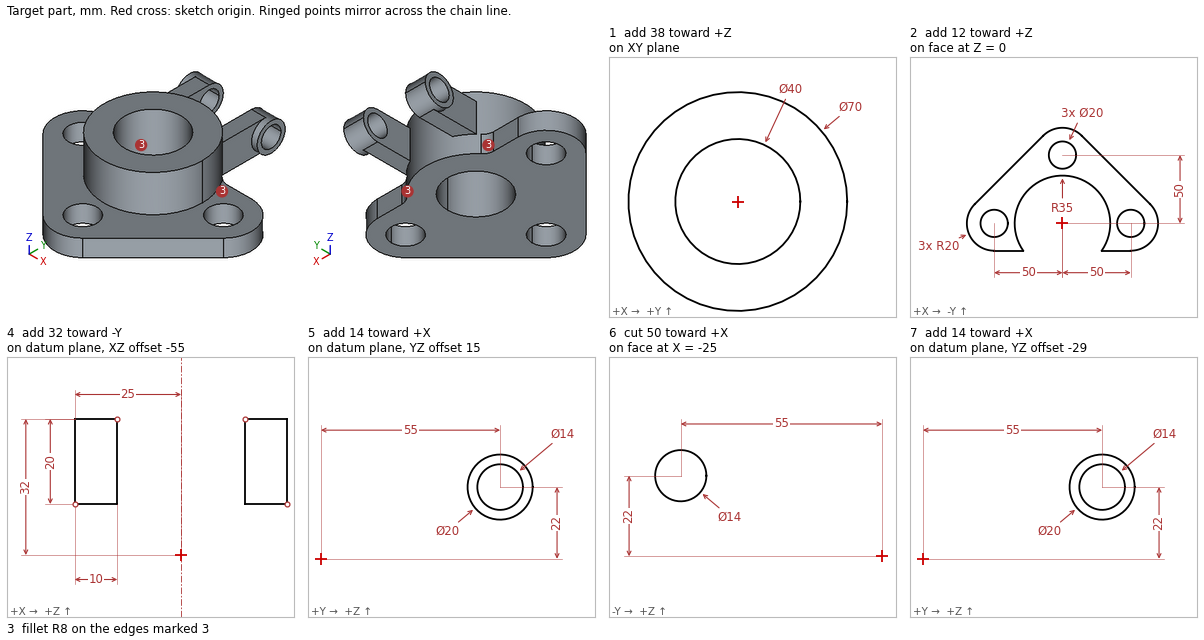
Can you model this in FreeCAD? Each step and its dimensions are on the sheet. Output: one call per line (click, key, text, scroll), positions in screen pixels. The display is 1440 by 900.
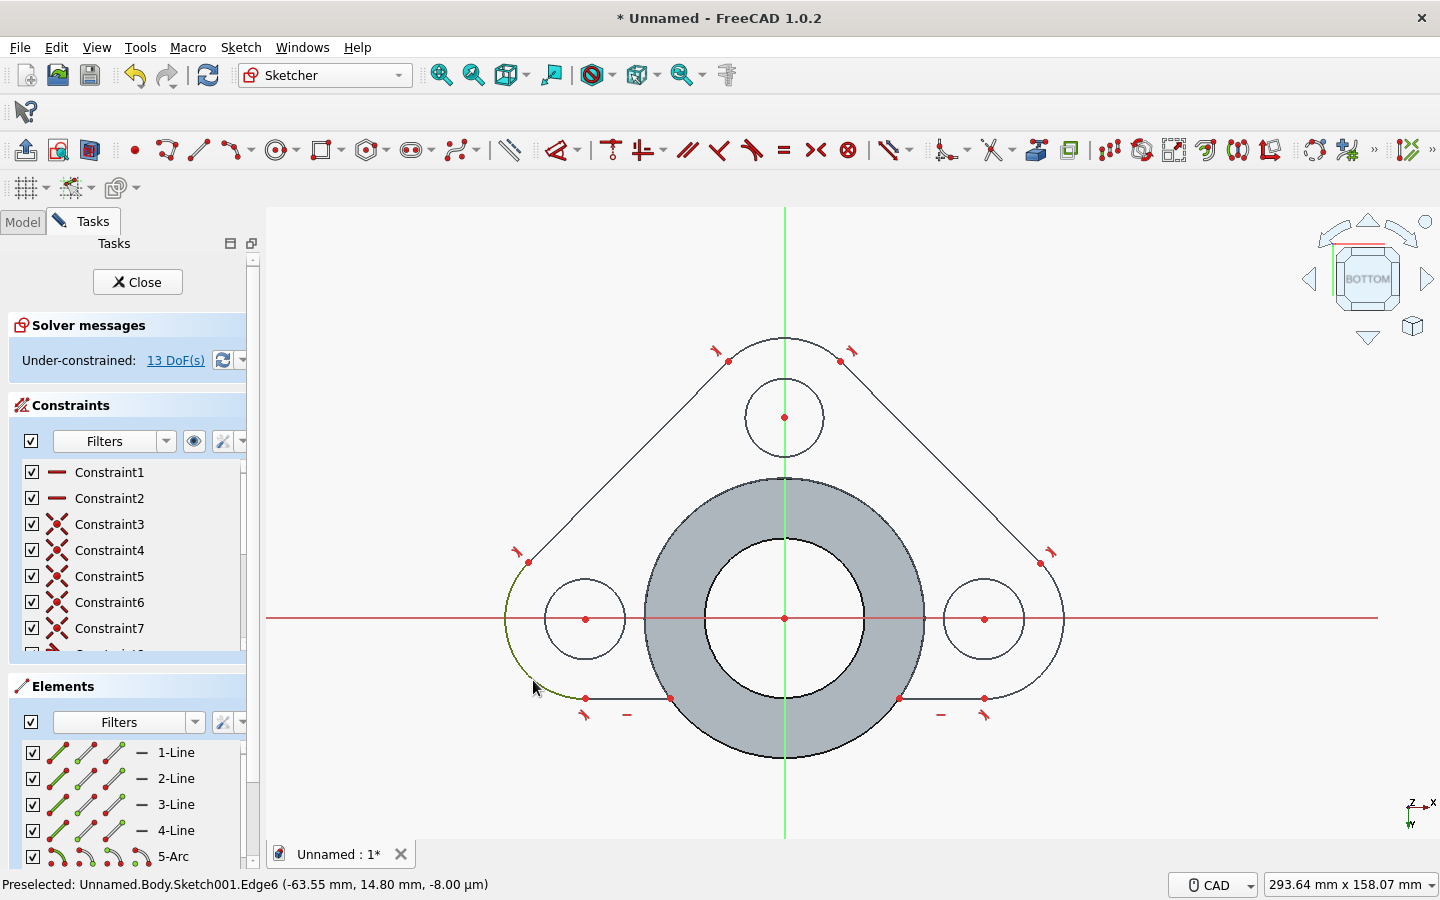
click(809, 342)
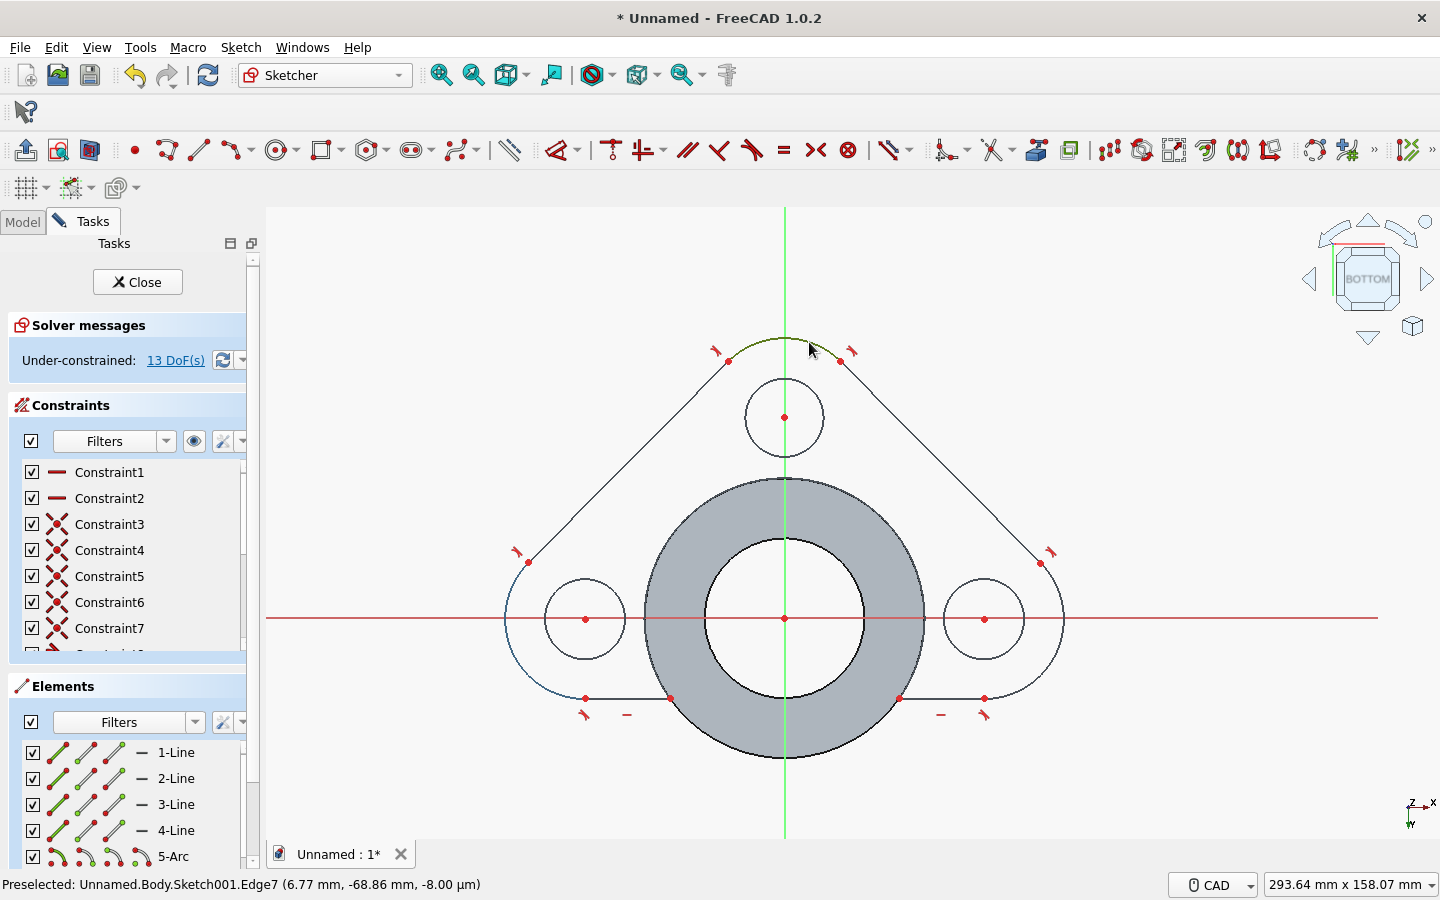
click(1036, 680)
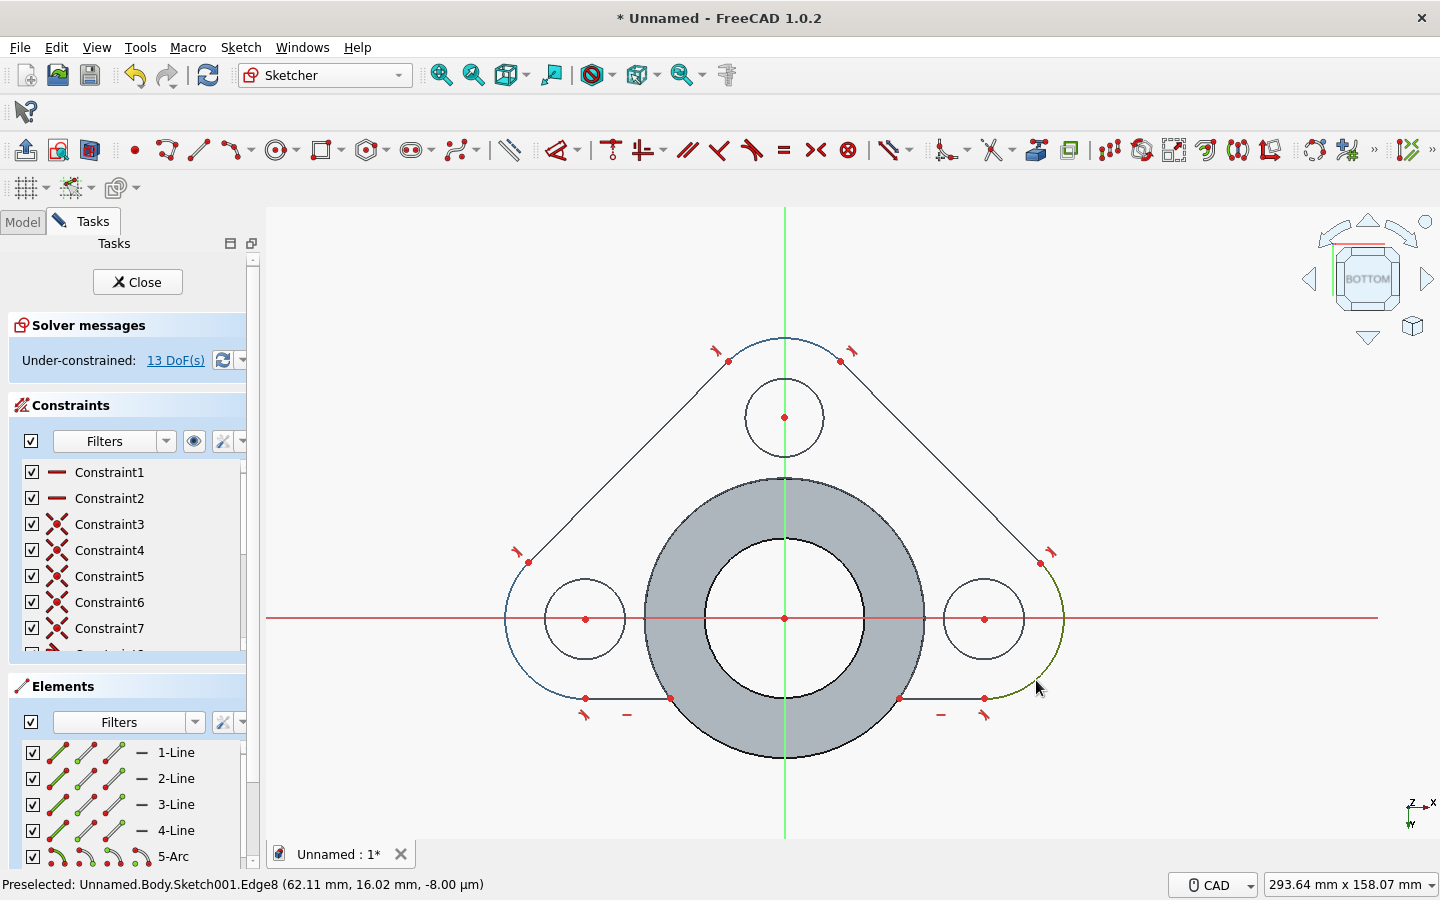
click(784, 150)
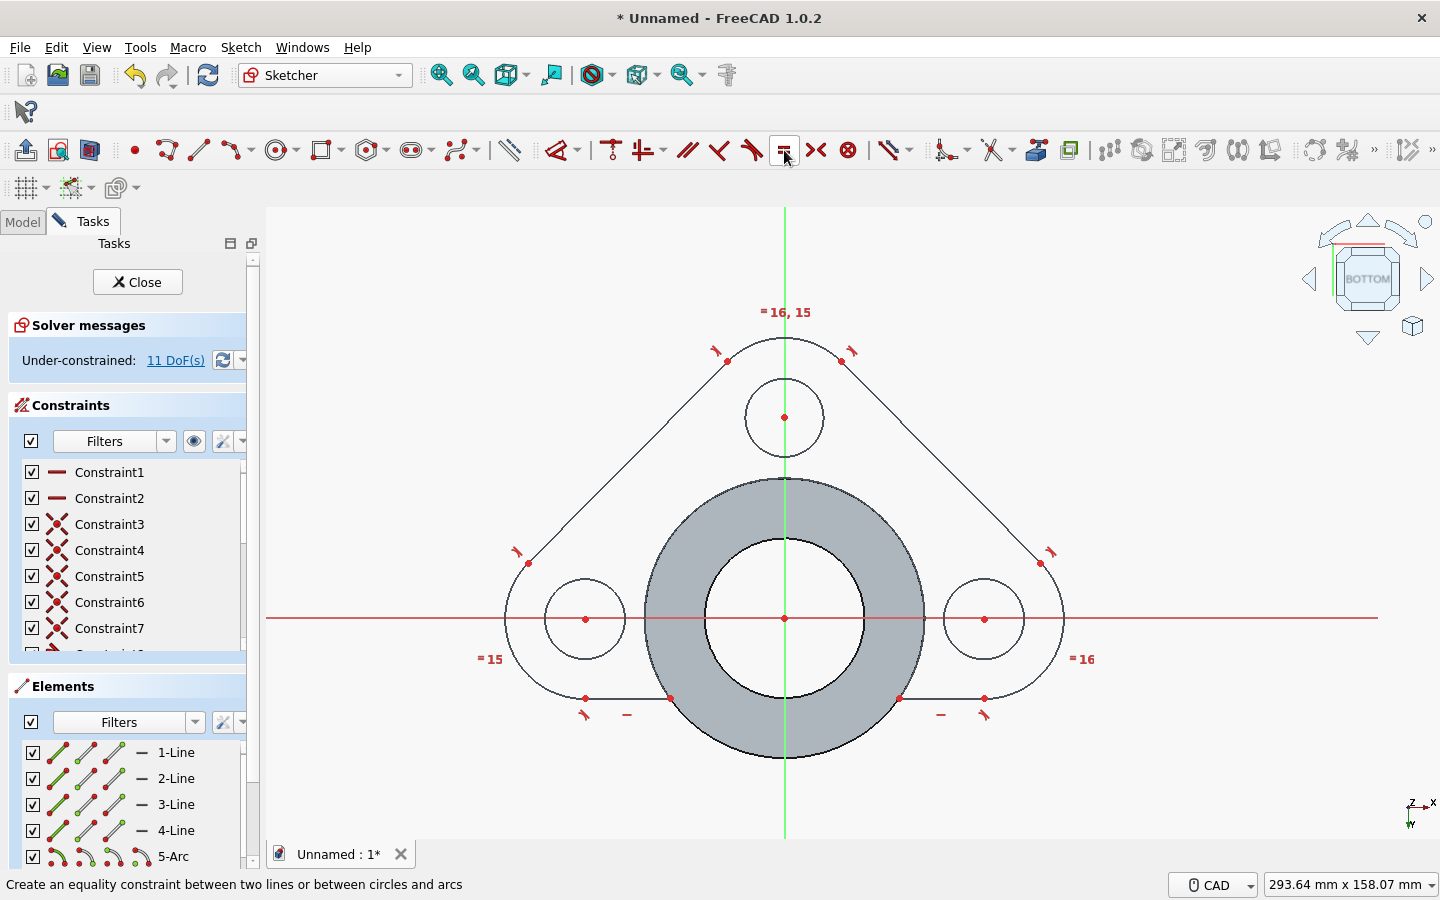
click(812, 390)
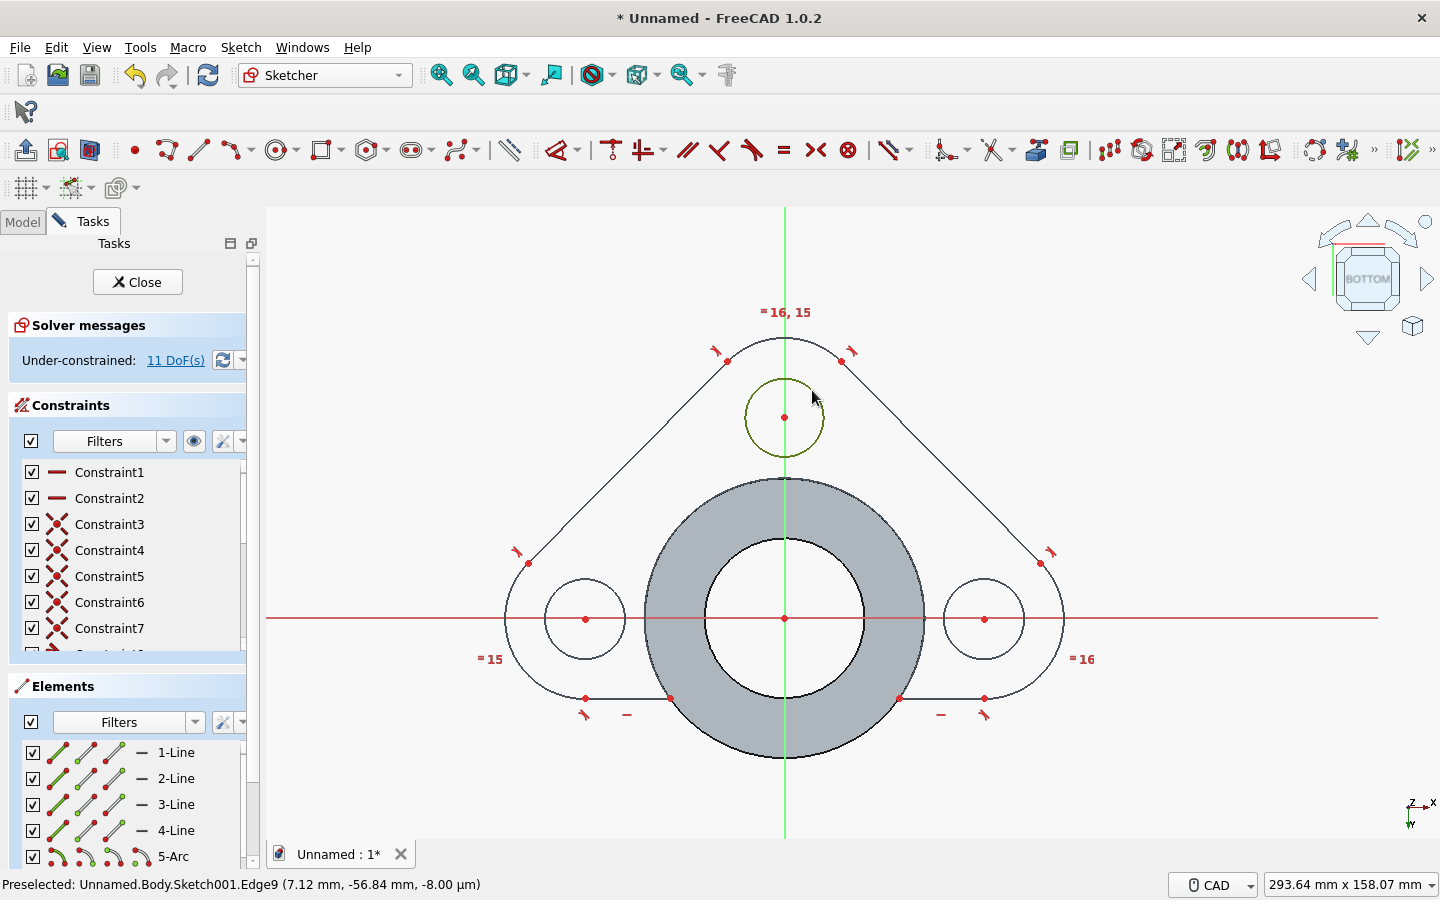
click(613, 591)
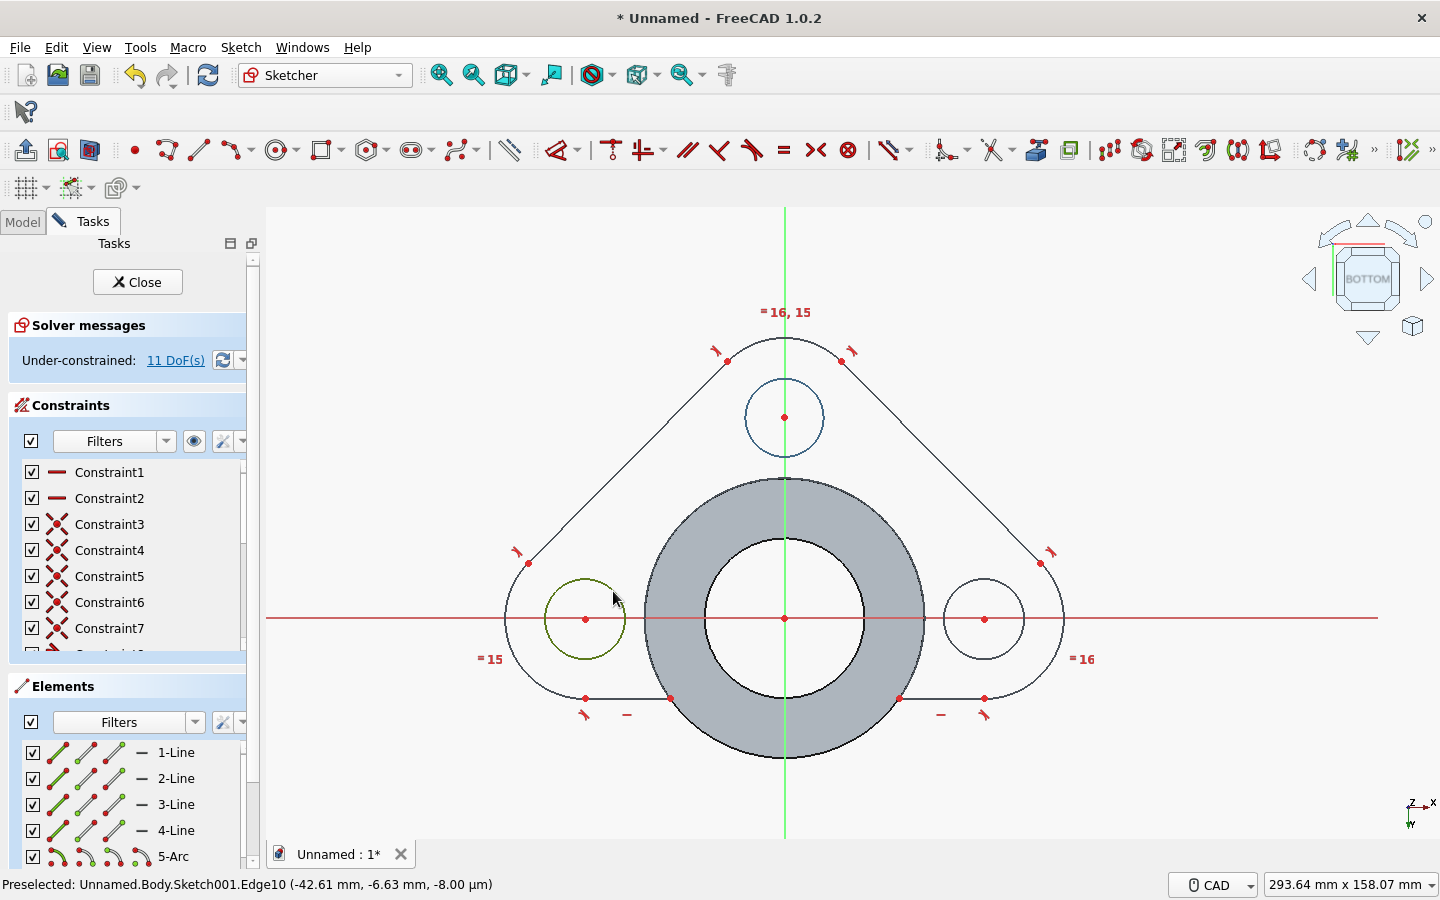
click(1012, 591)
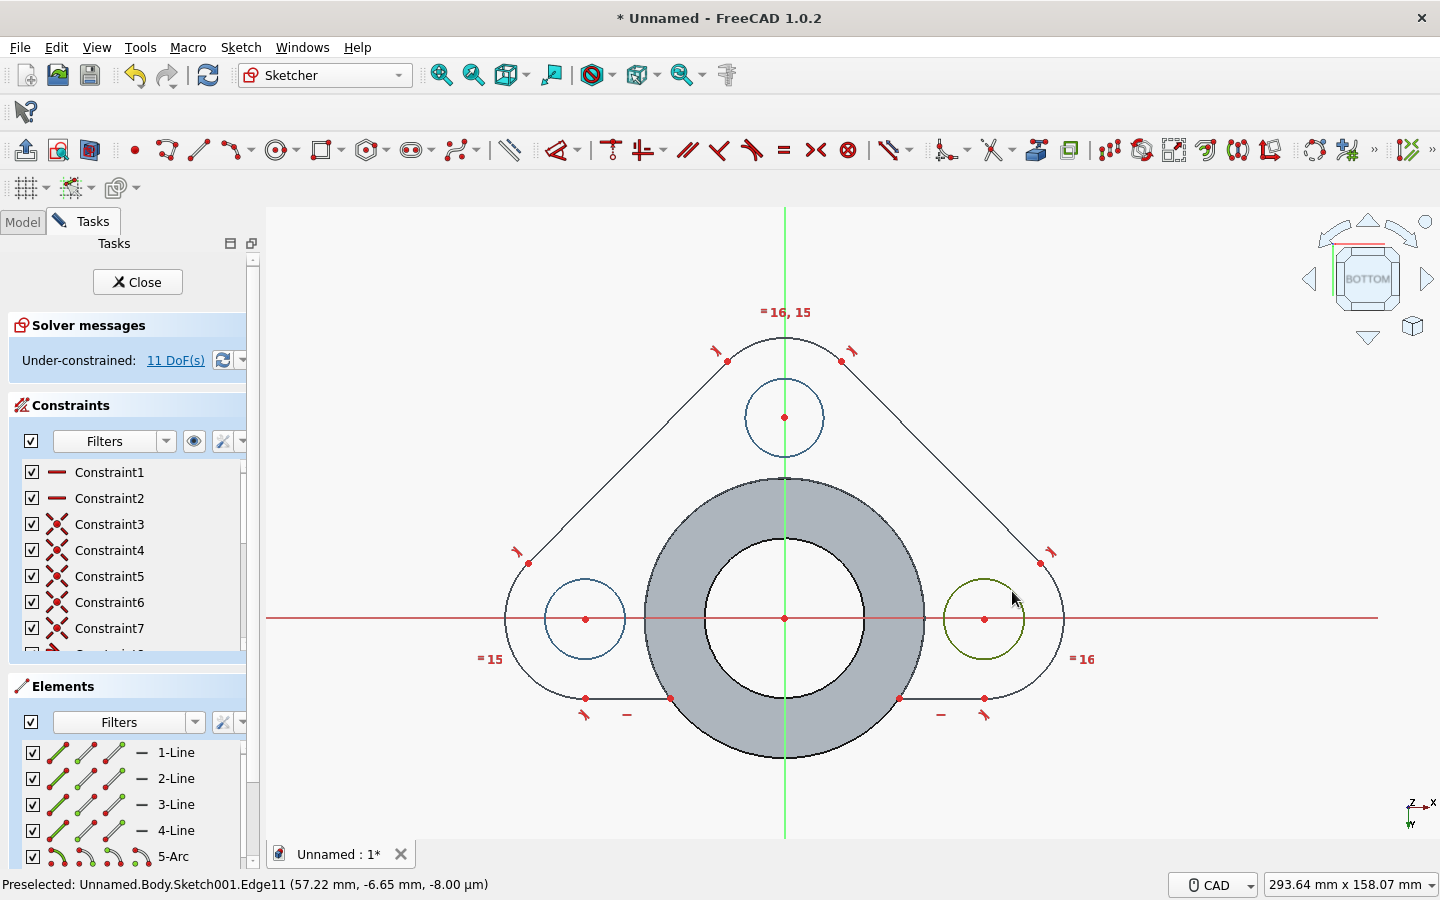
click(784, 150)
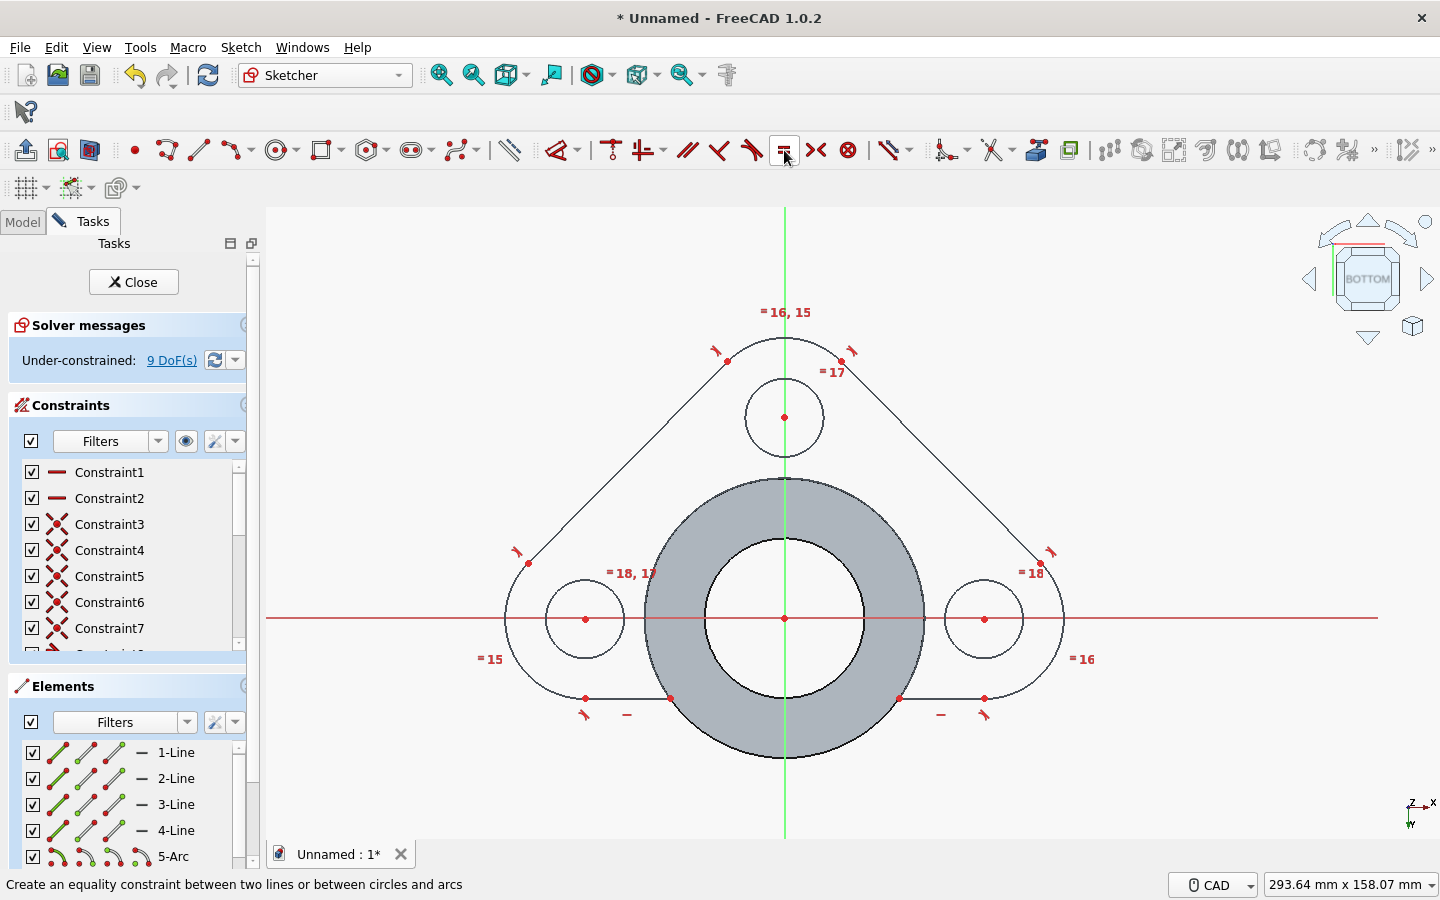
click(585, 619)